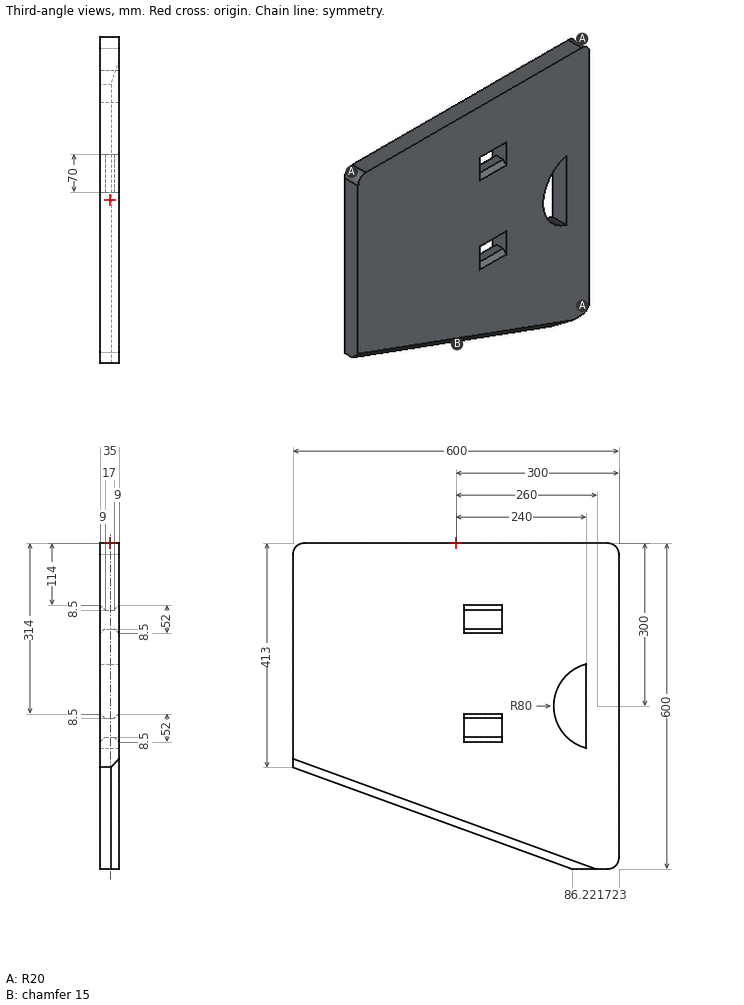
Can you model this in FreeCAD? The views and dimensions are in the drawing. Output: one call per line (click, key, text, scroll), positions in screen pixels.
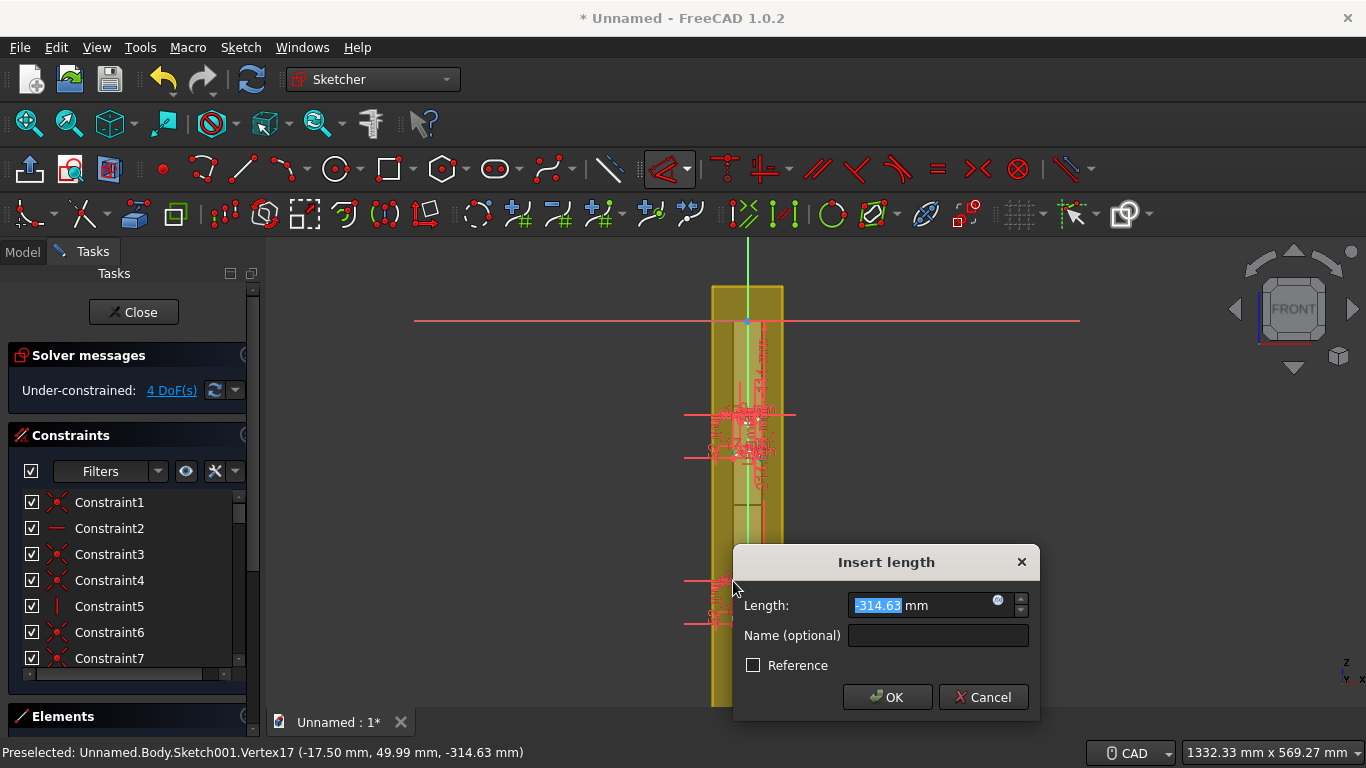
text(-314)
key(Return)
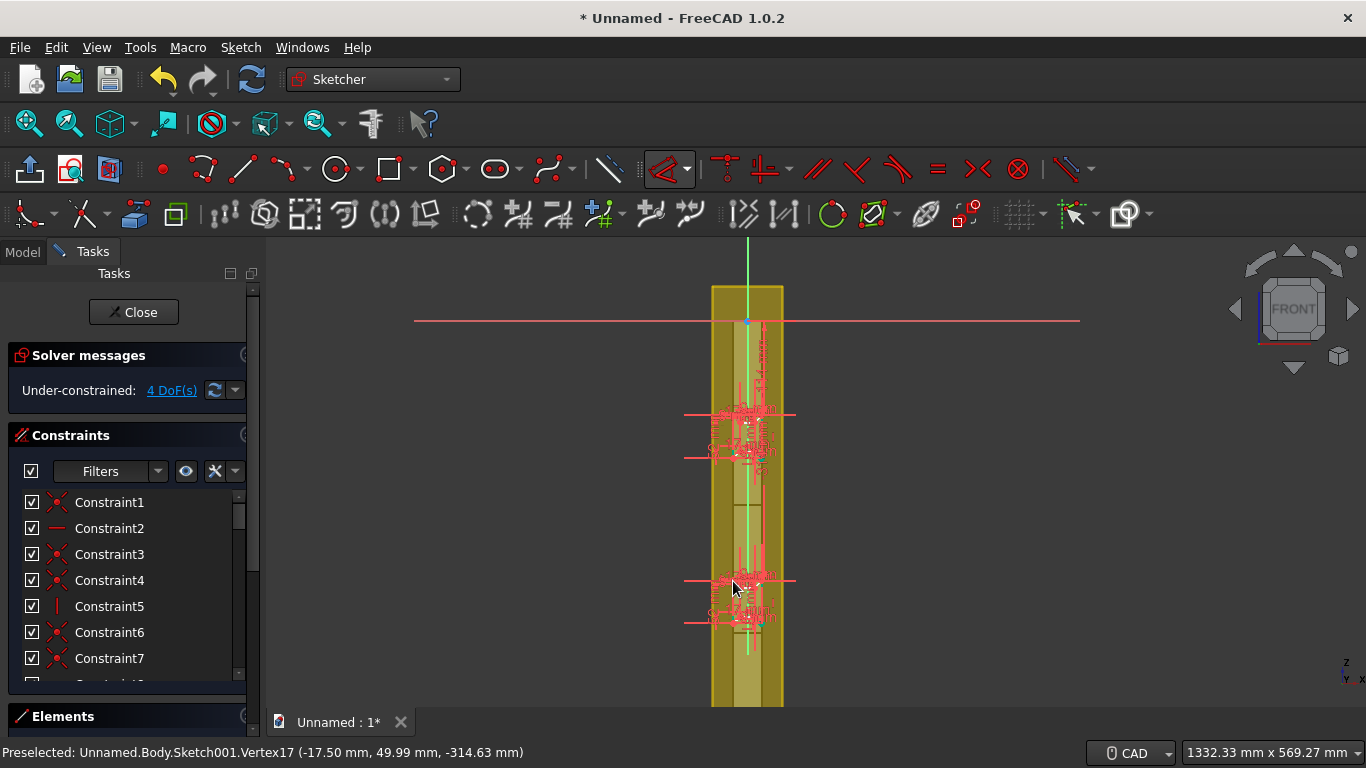
scroll(738, 420, up, 9)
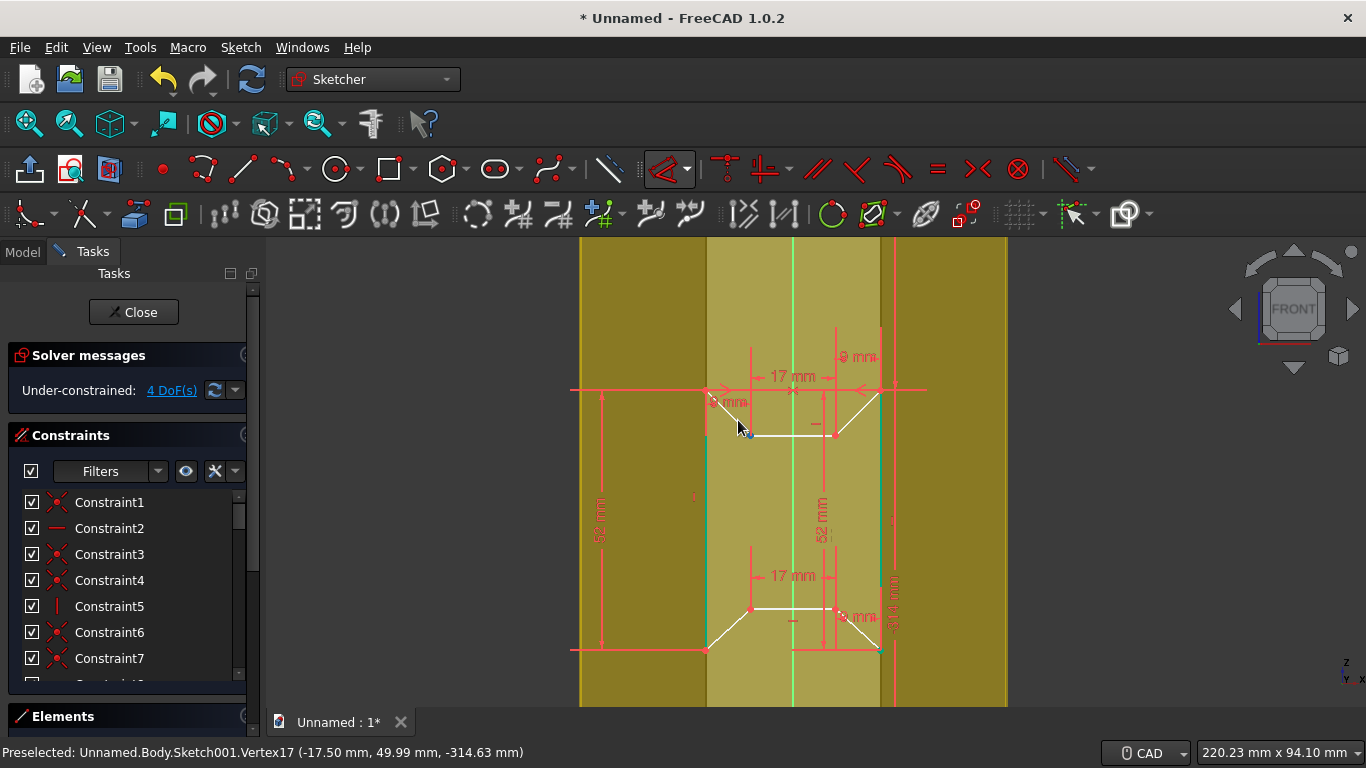
click(733, 417)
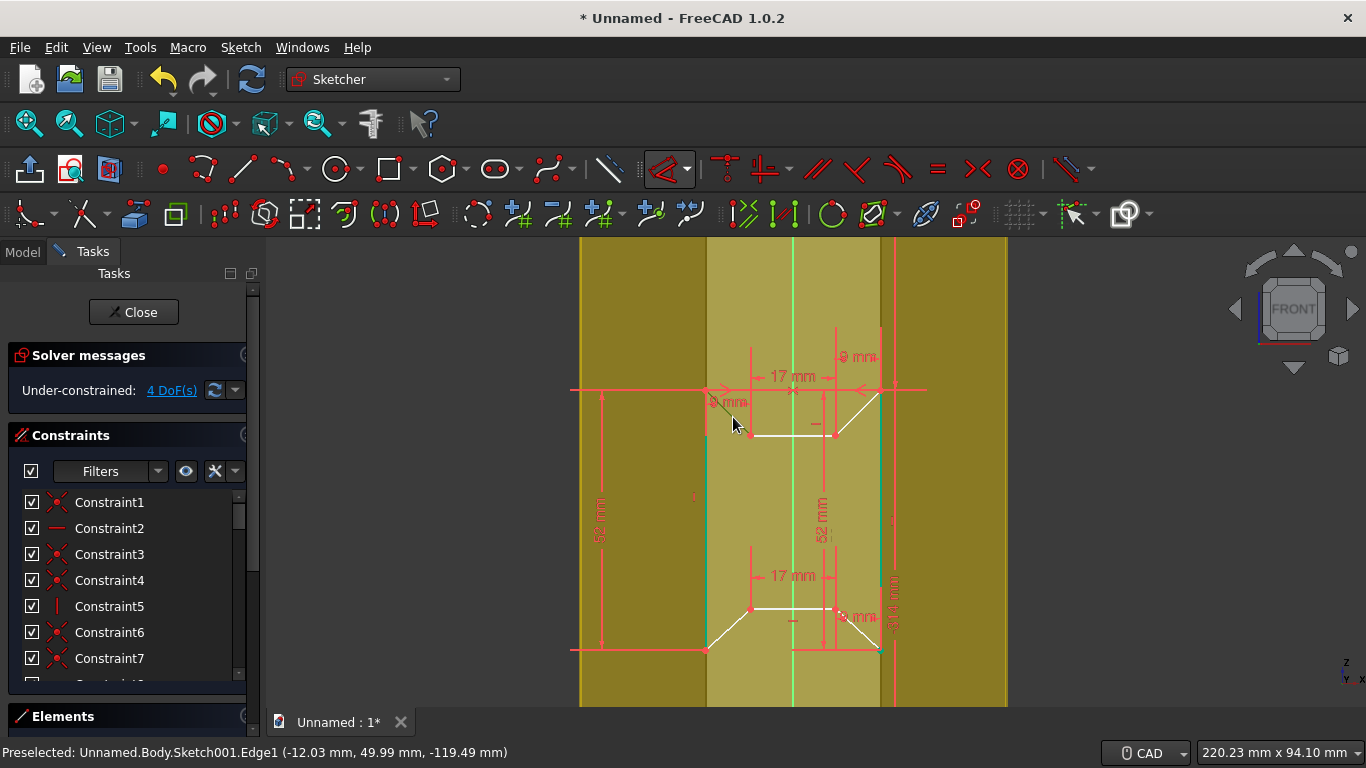
click(690, 170)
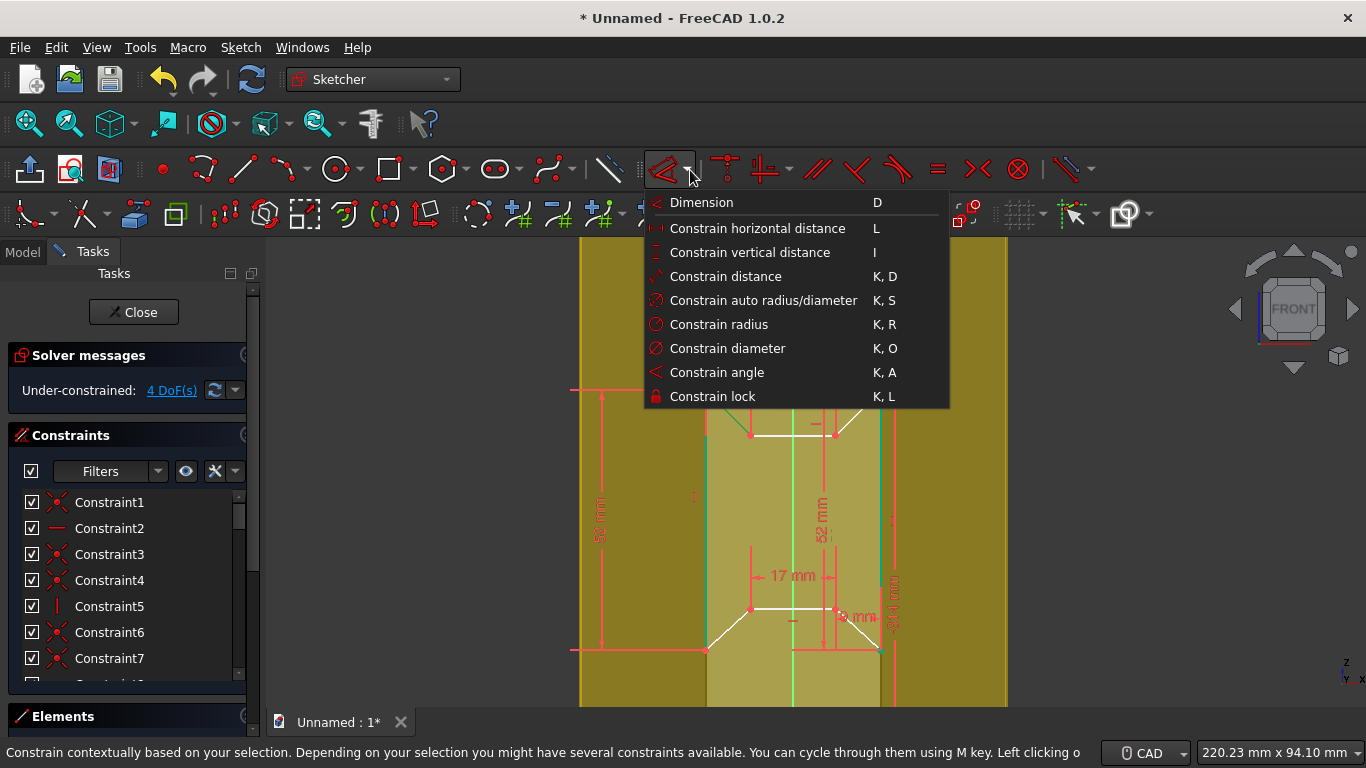
click(797, 252)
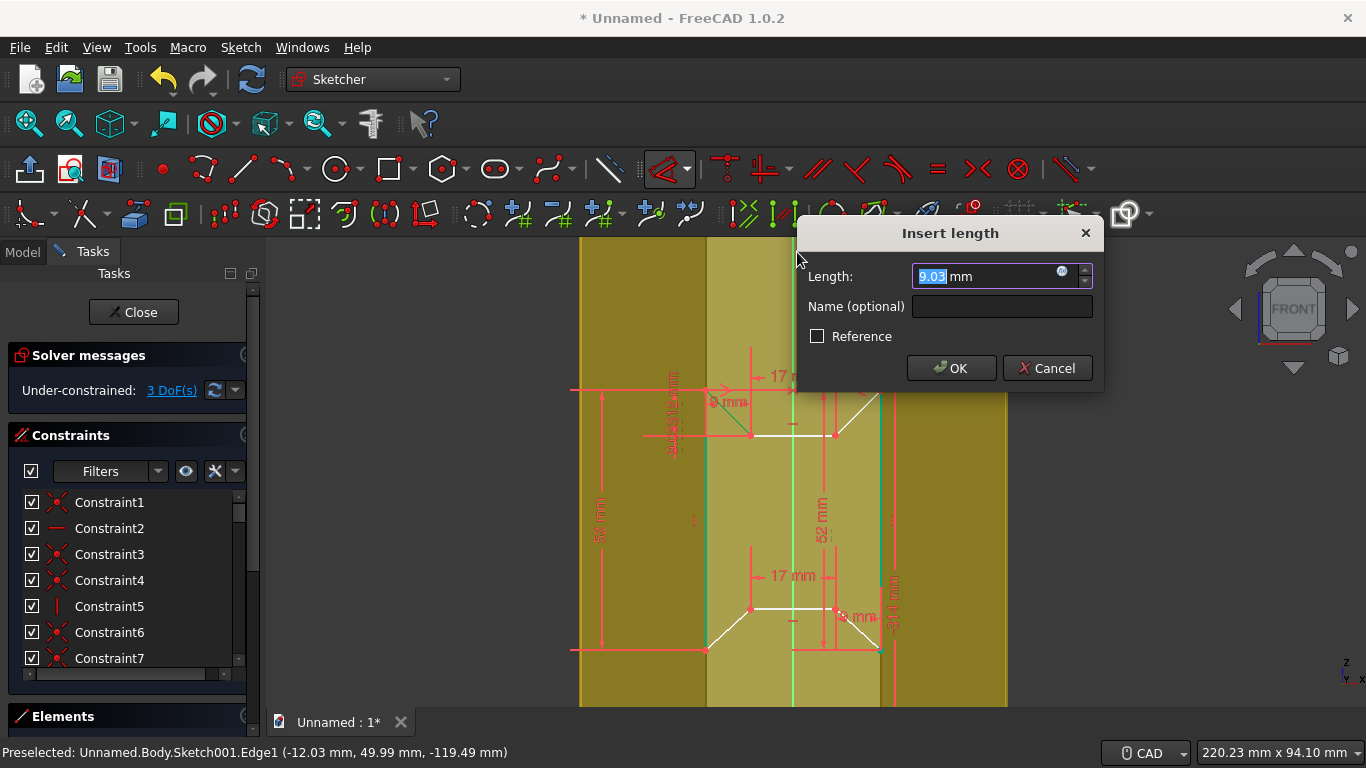
text(8.5)
key(Return)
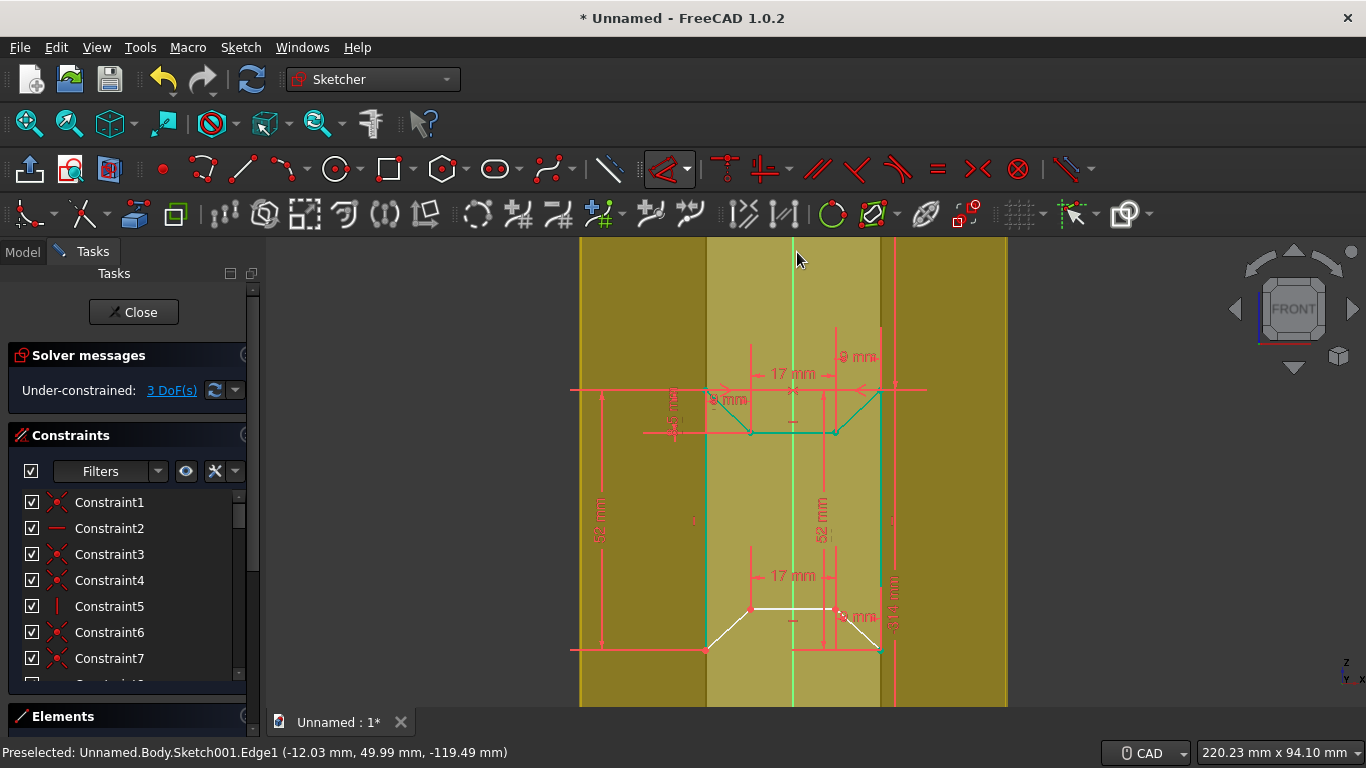
click(867, 638)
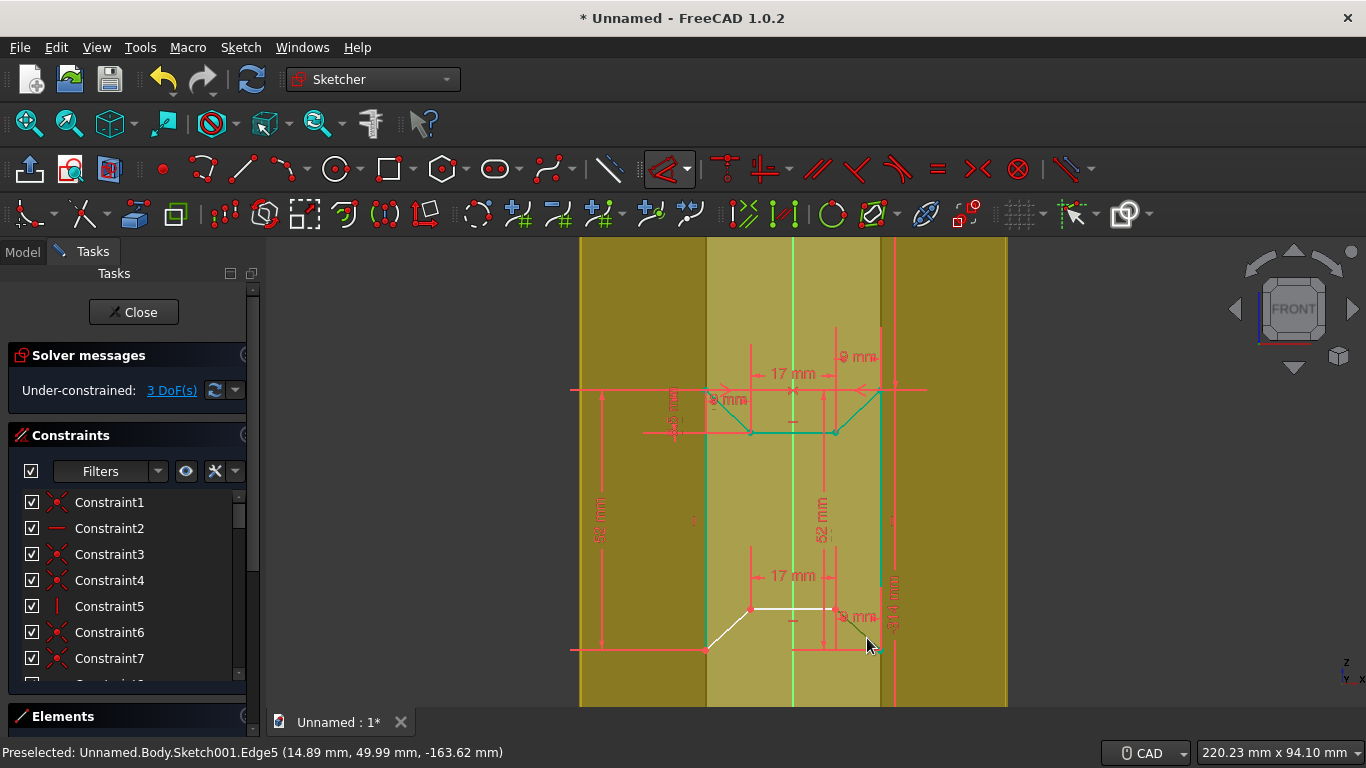
key(i)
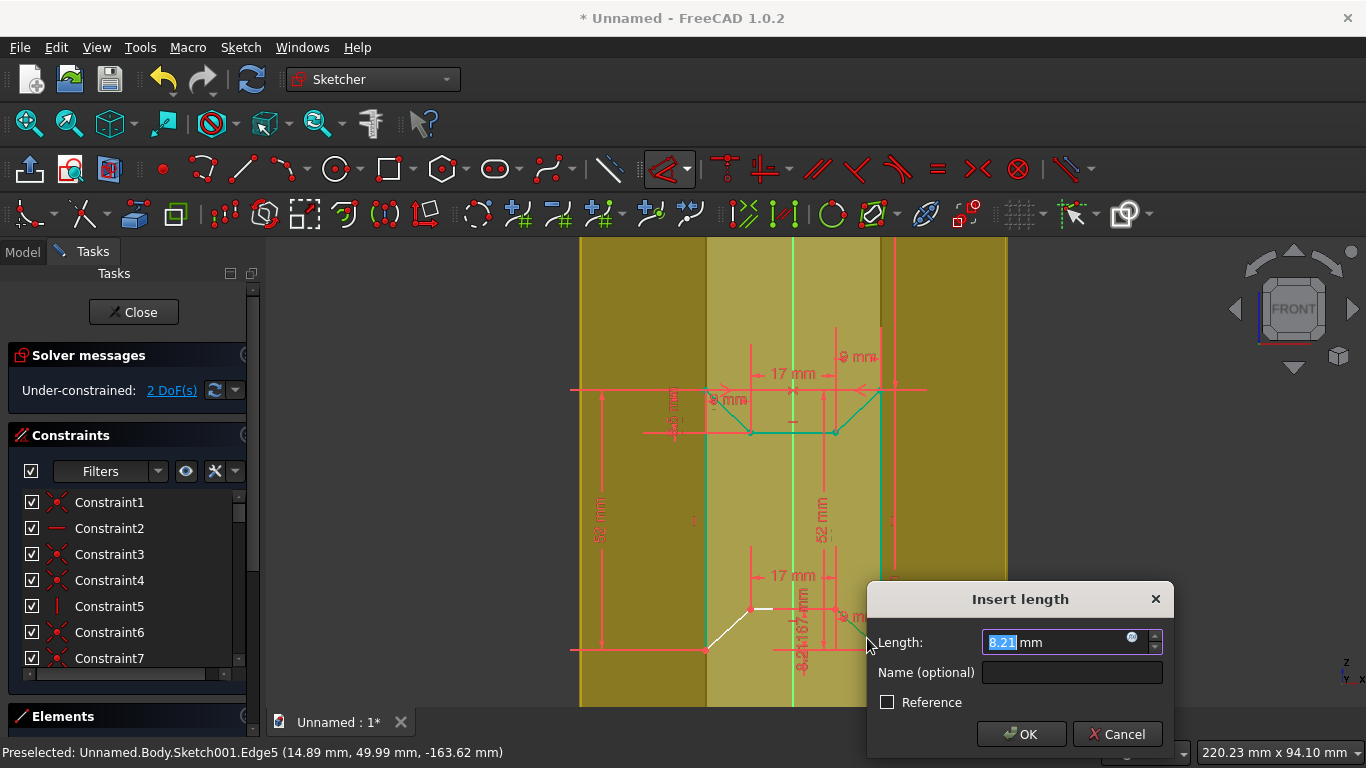
text(8.5)
key(Return)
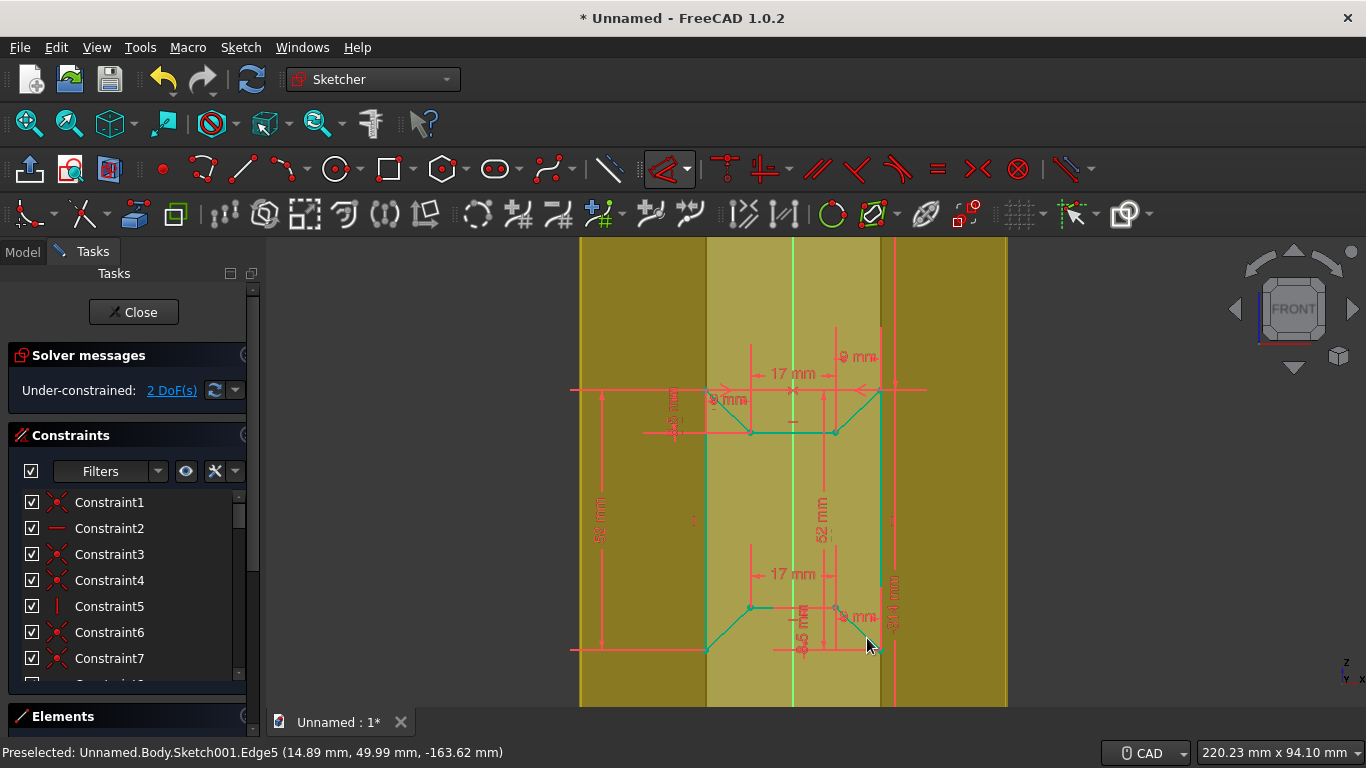
scroll(738, 420, down, 9)